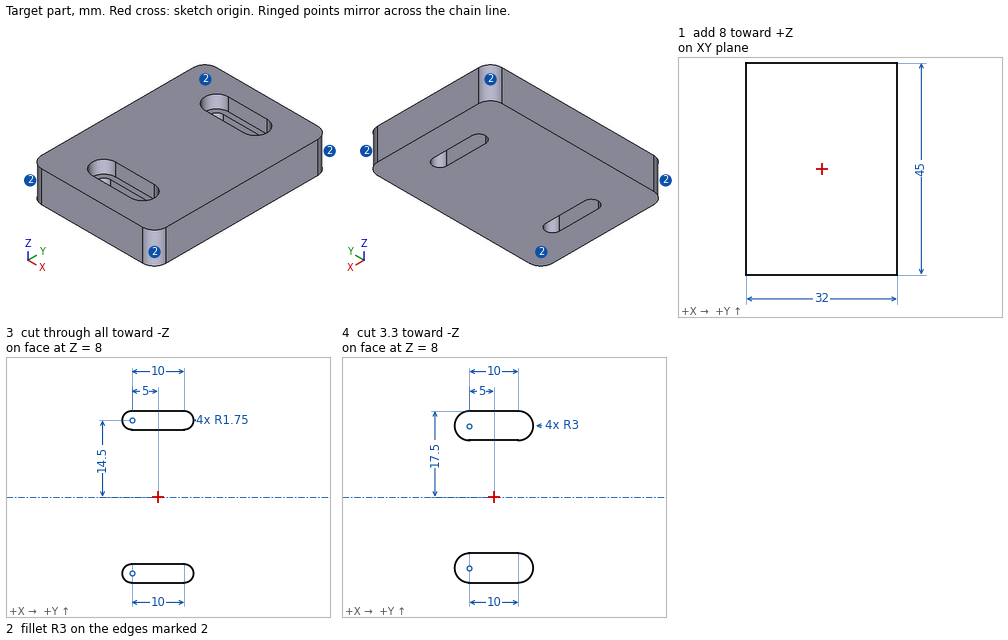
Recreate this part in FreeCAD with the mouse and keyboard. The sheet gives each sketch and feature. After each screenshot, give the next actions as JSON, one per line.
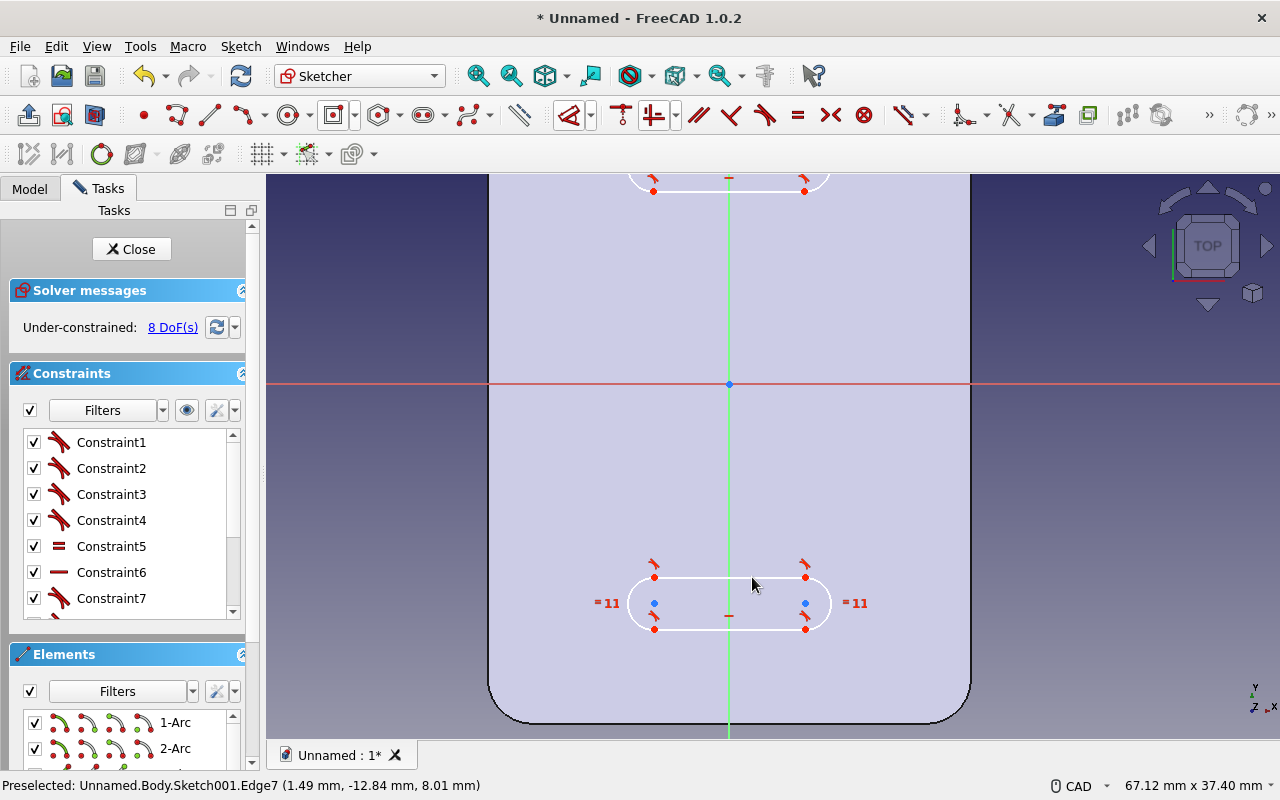
{"action": "scroll", "coordinate": [654, 604], "scroll_direction": "down", "scroll_amount": 2}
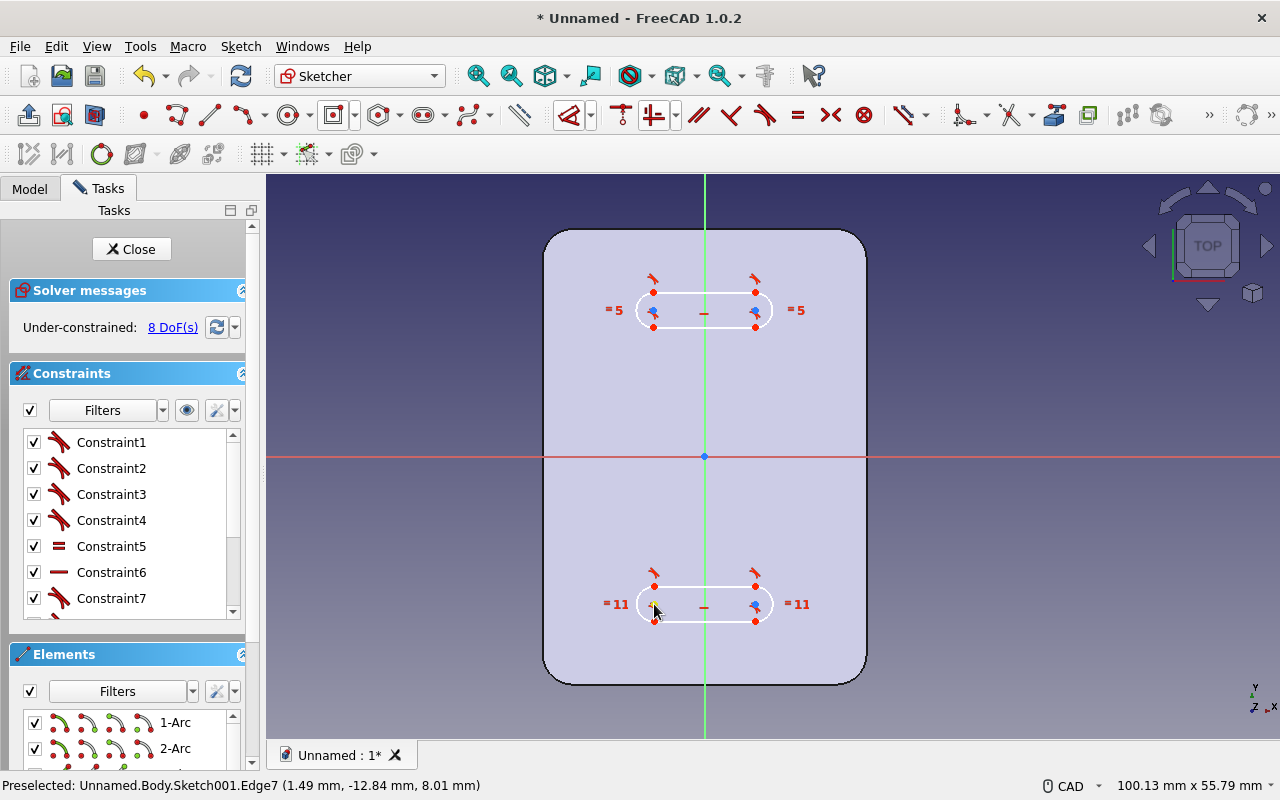
{"action": "left_click", "coordinate": [640, 300]}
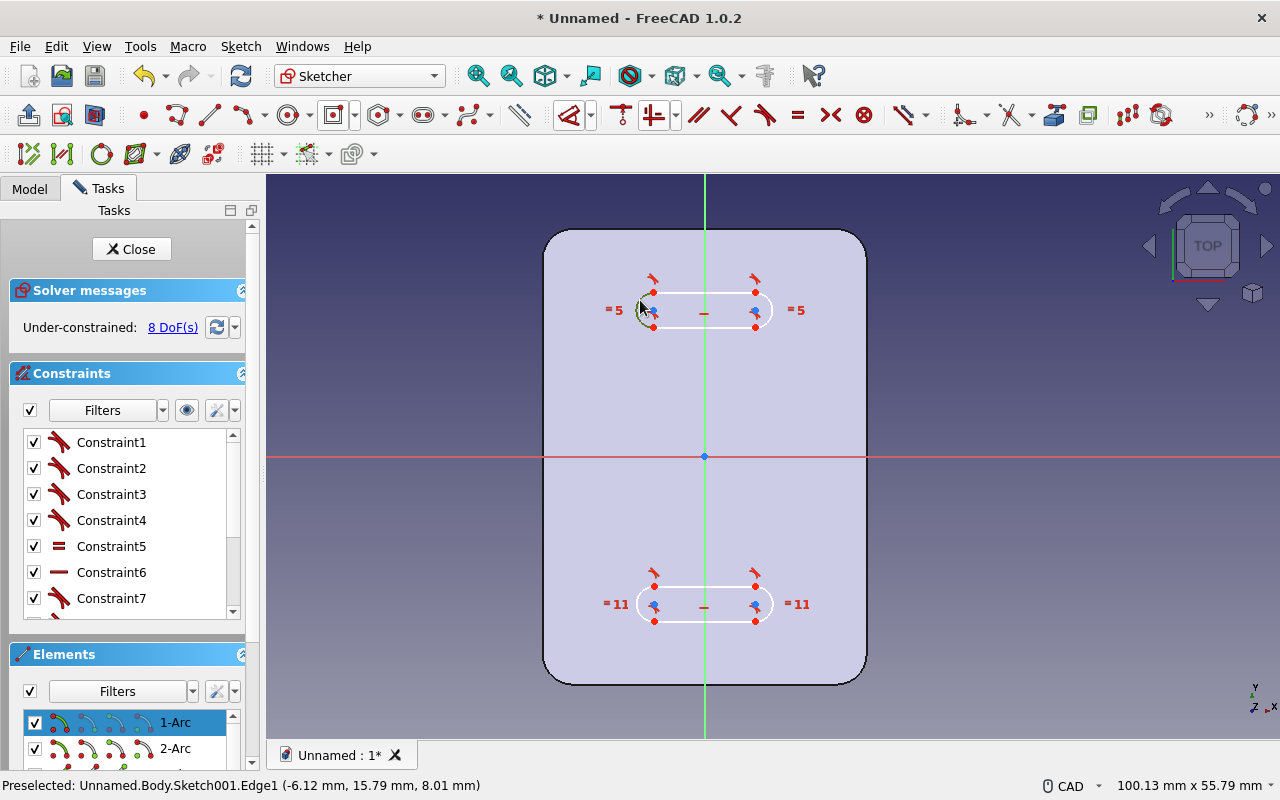
{"action": "left_click", "coordinate": [640, 594]}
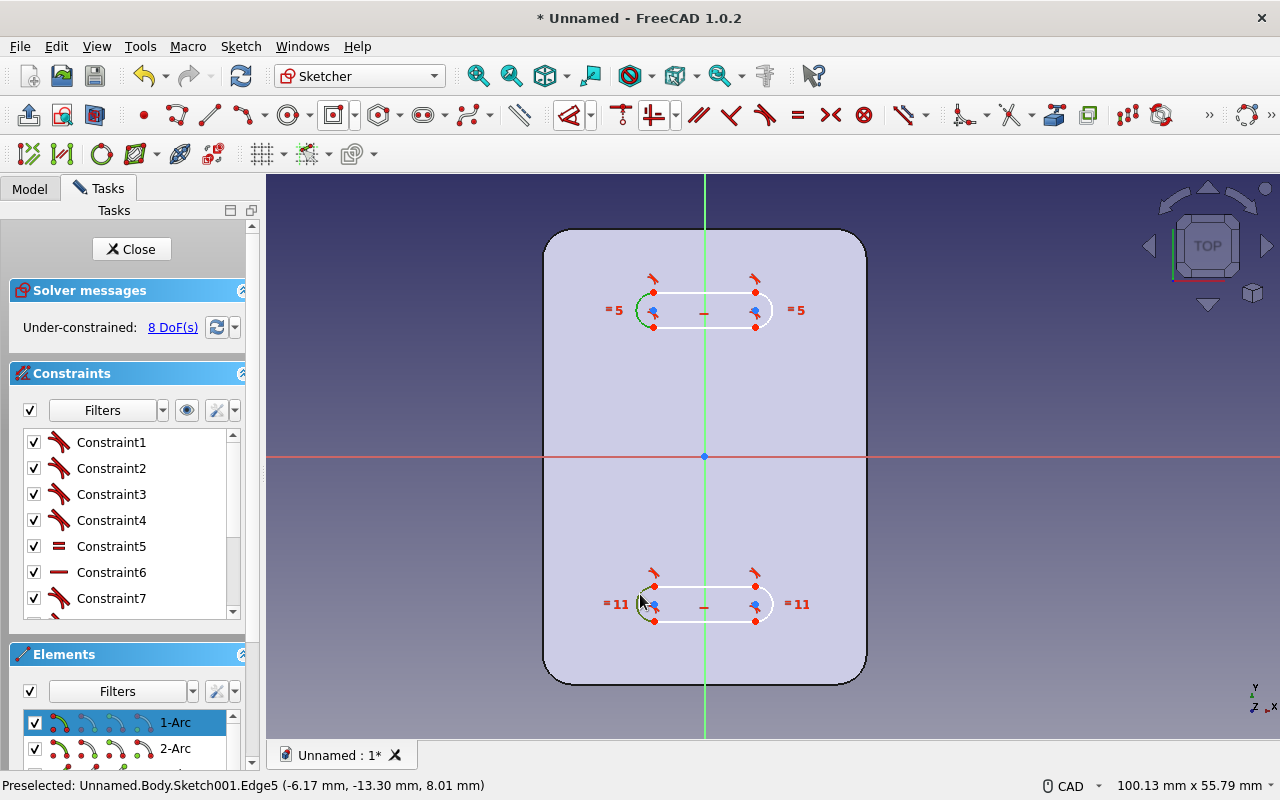
{"action": "left_click", "coordinate": [798, 116]}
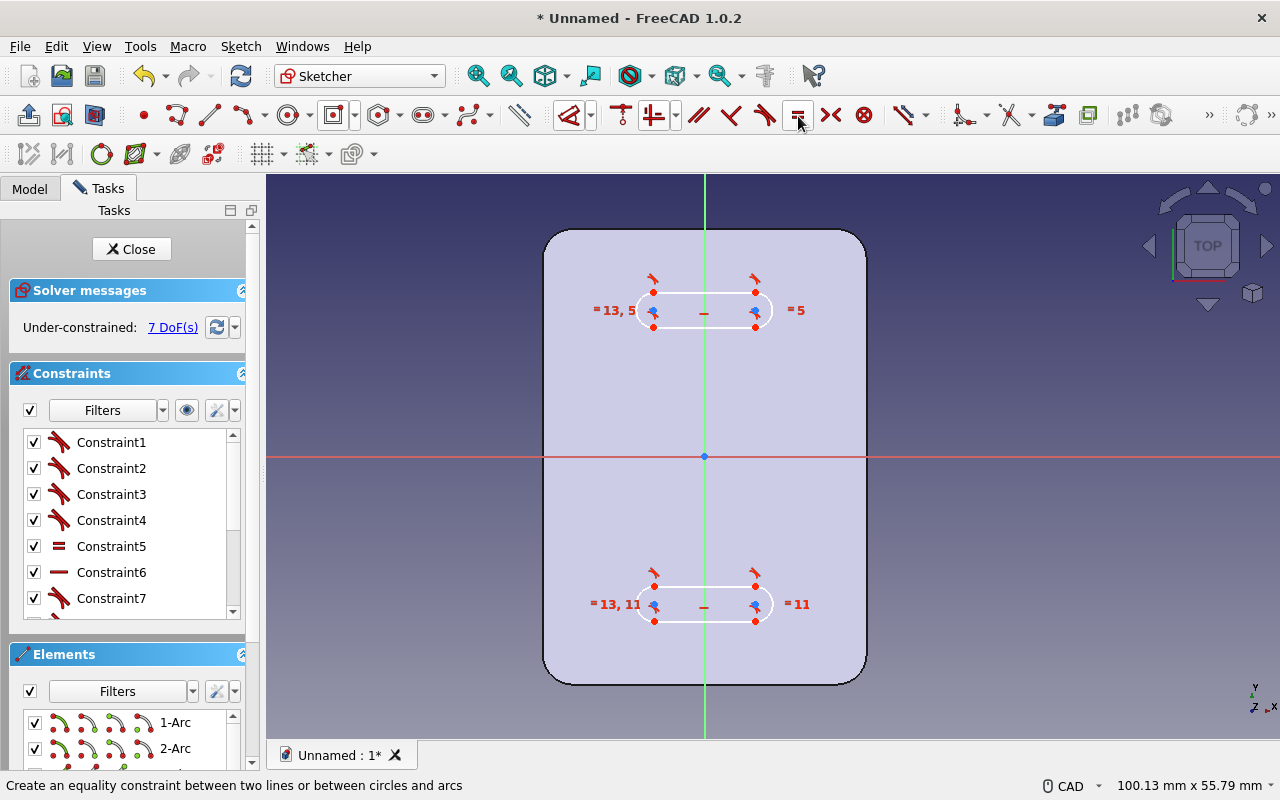
{"action": "left_click", "coordinate": [654, 310]}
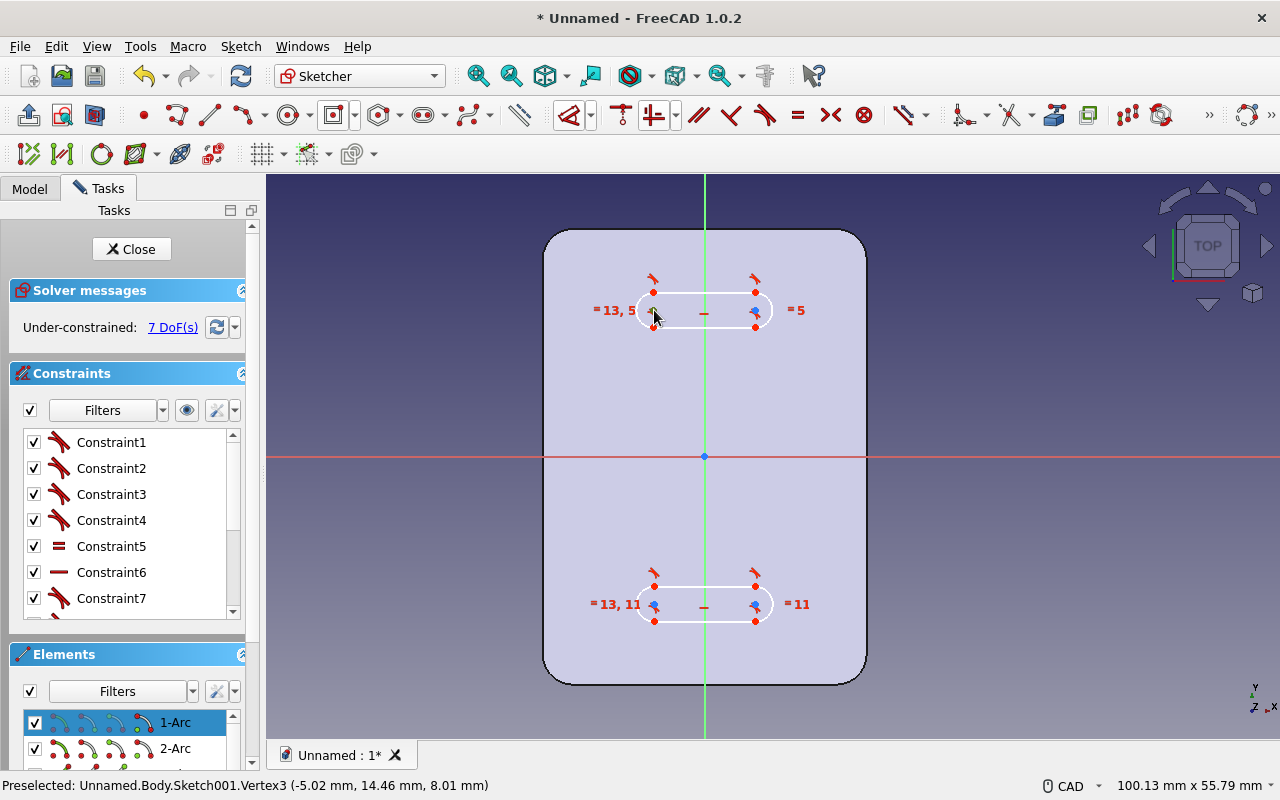
{"action": "left_click", "coordinate": [654, 604]}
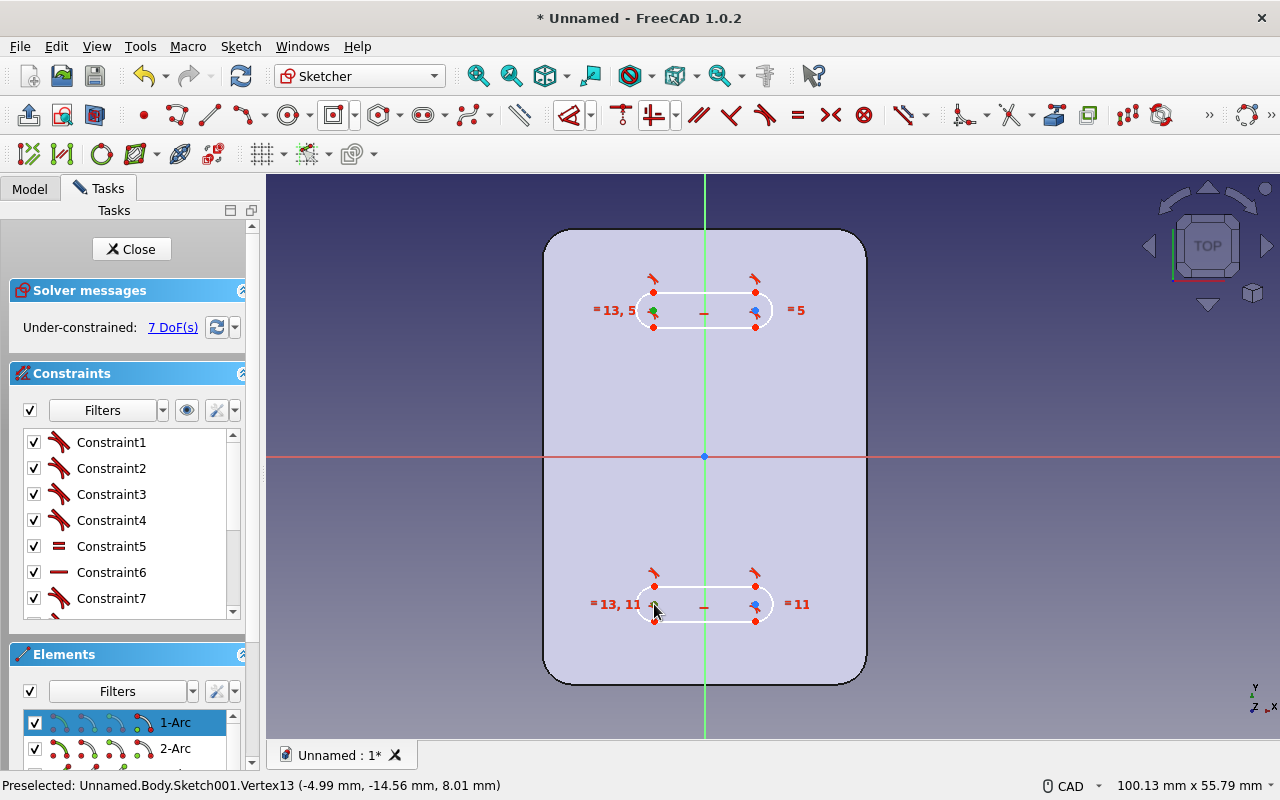
{"action": "left_click", "coordinate": [353, 457]}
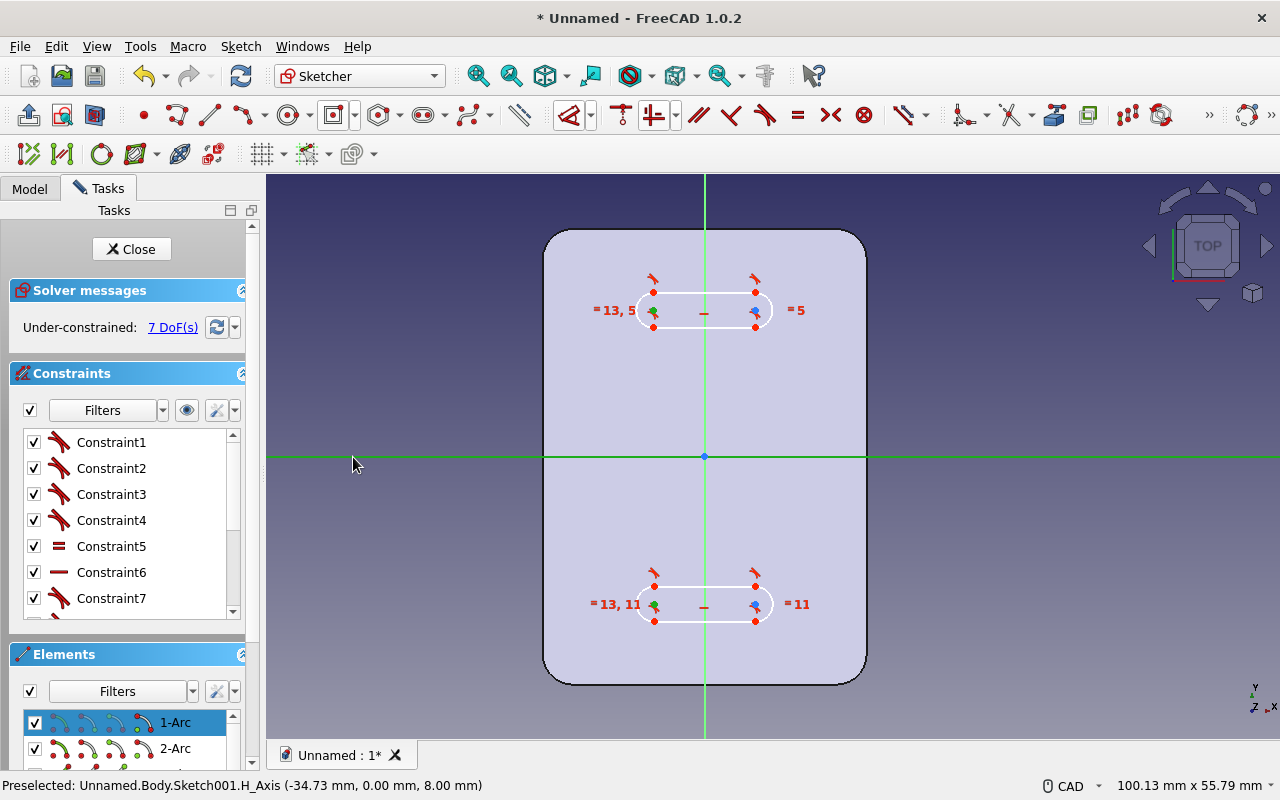
{"action": "left_click", "coordinate": [831, 116]}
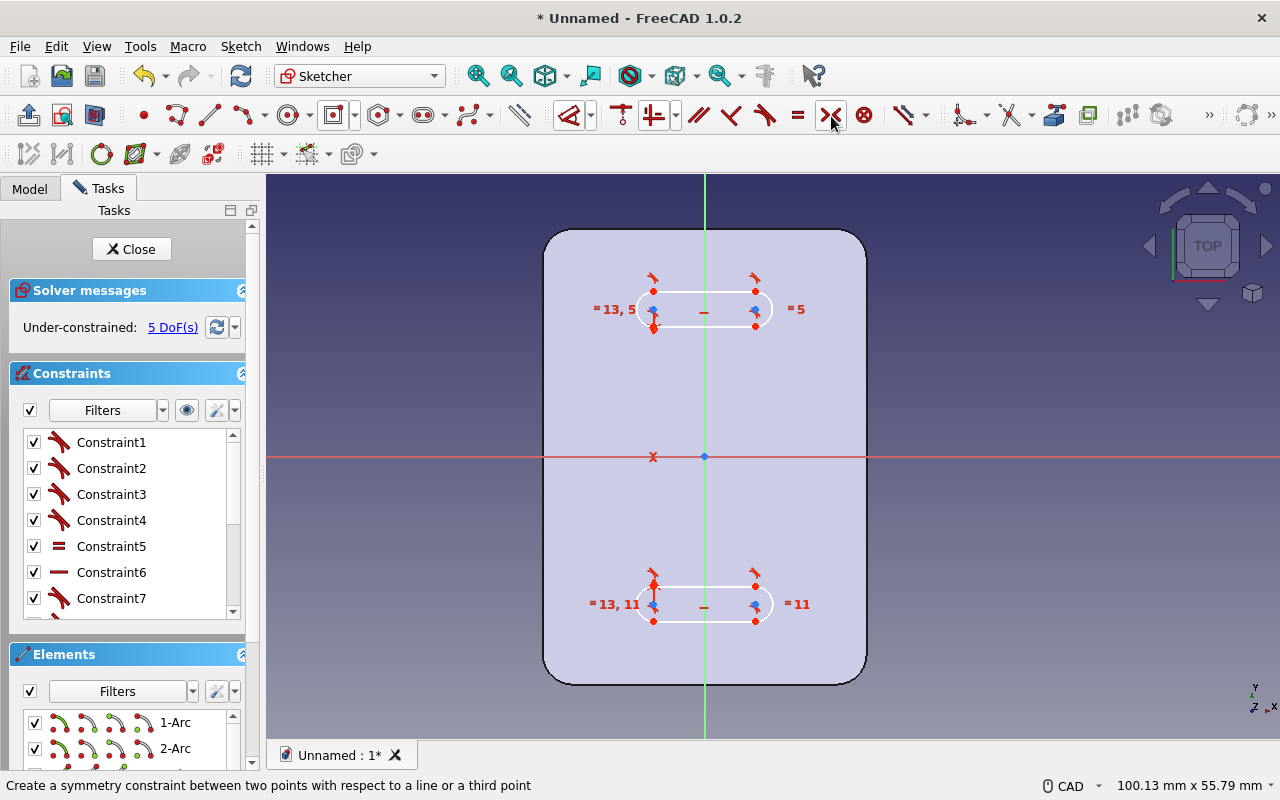
{"action": "scroll", "coordinate": [640, 299], "scroll_direction": "up", "scroll_amount": 5}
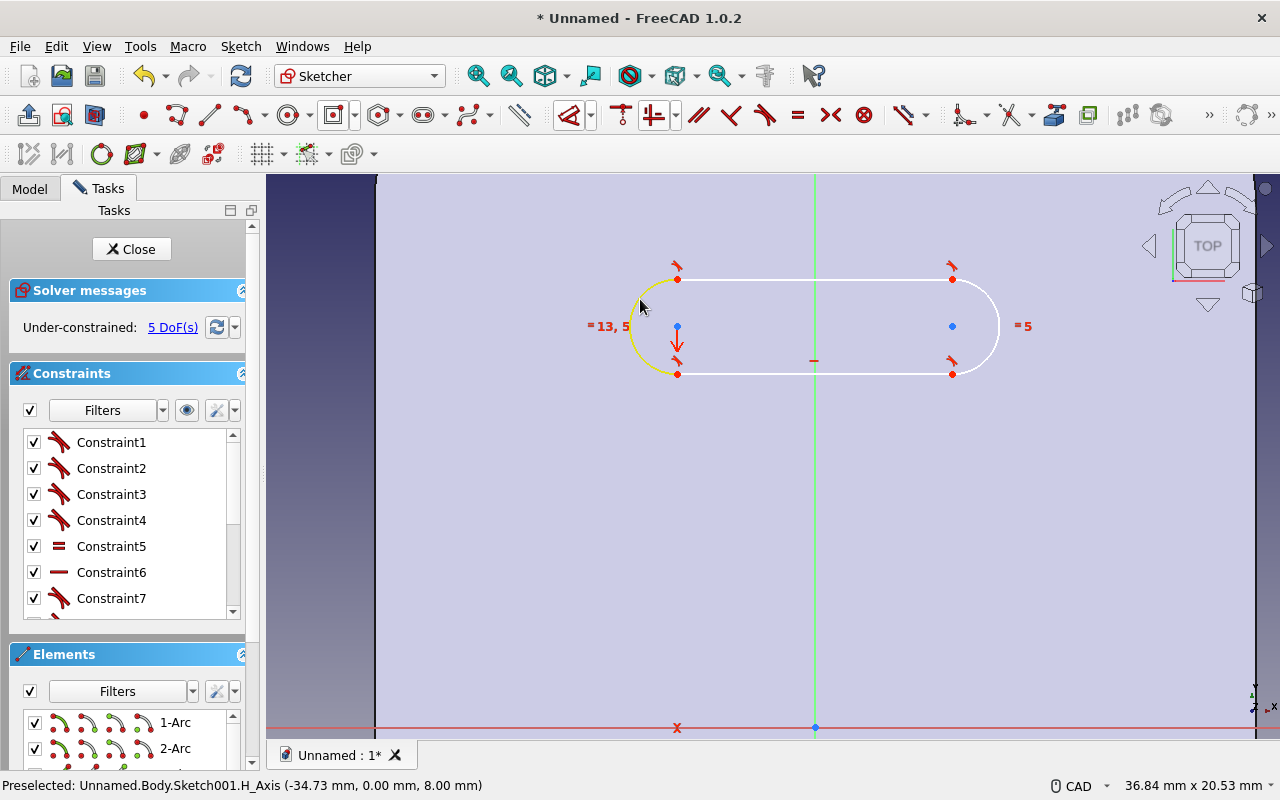
{"action": "left_click", "coordinate": [639, 299]}